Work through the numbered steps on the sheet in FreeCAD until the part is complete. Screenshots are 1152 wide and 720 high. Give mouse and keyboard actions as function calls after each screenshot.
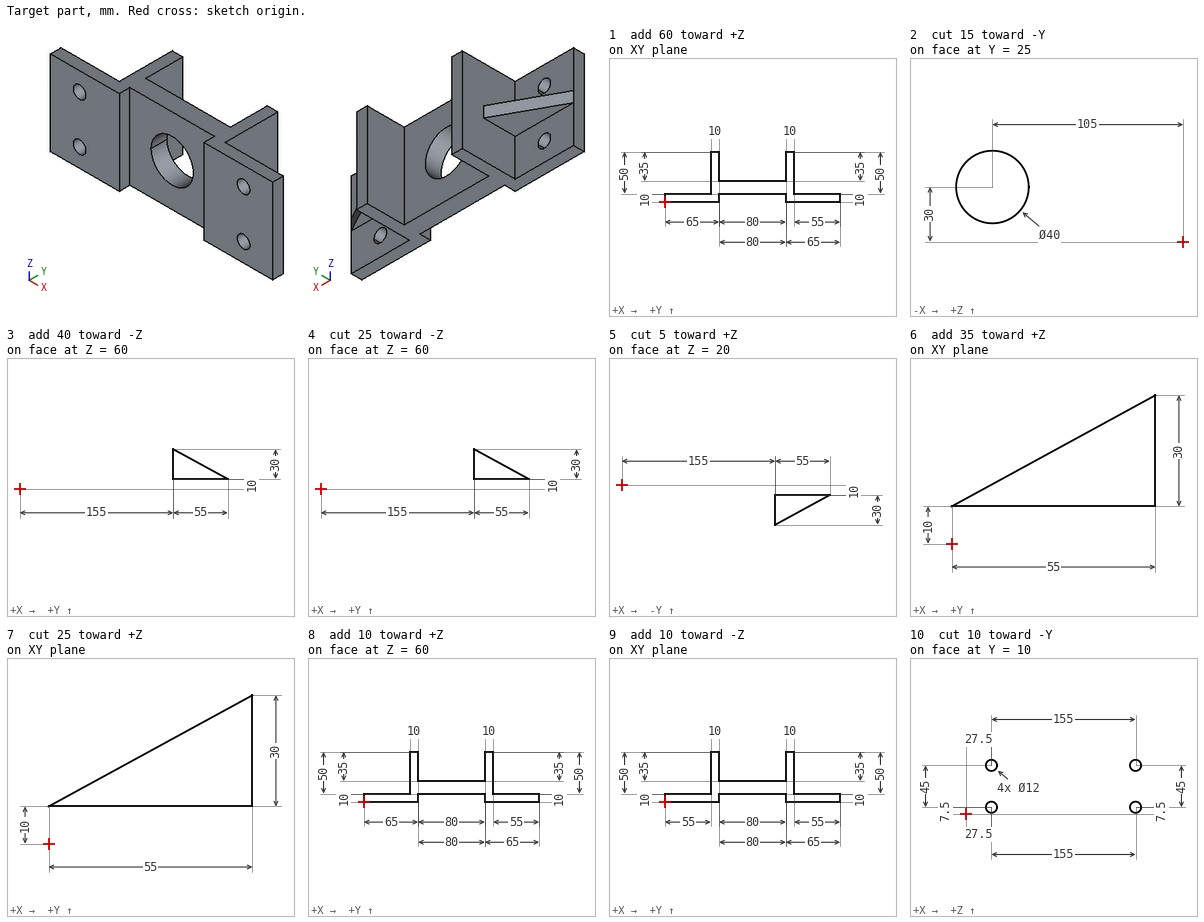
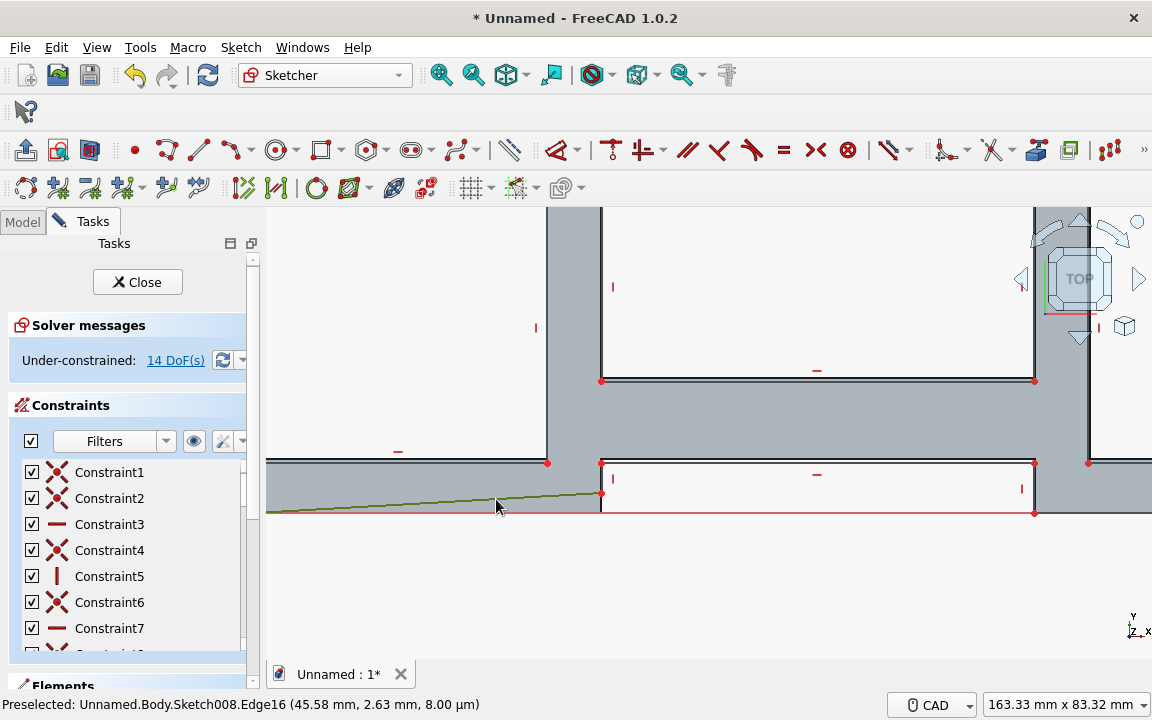
key(h)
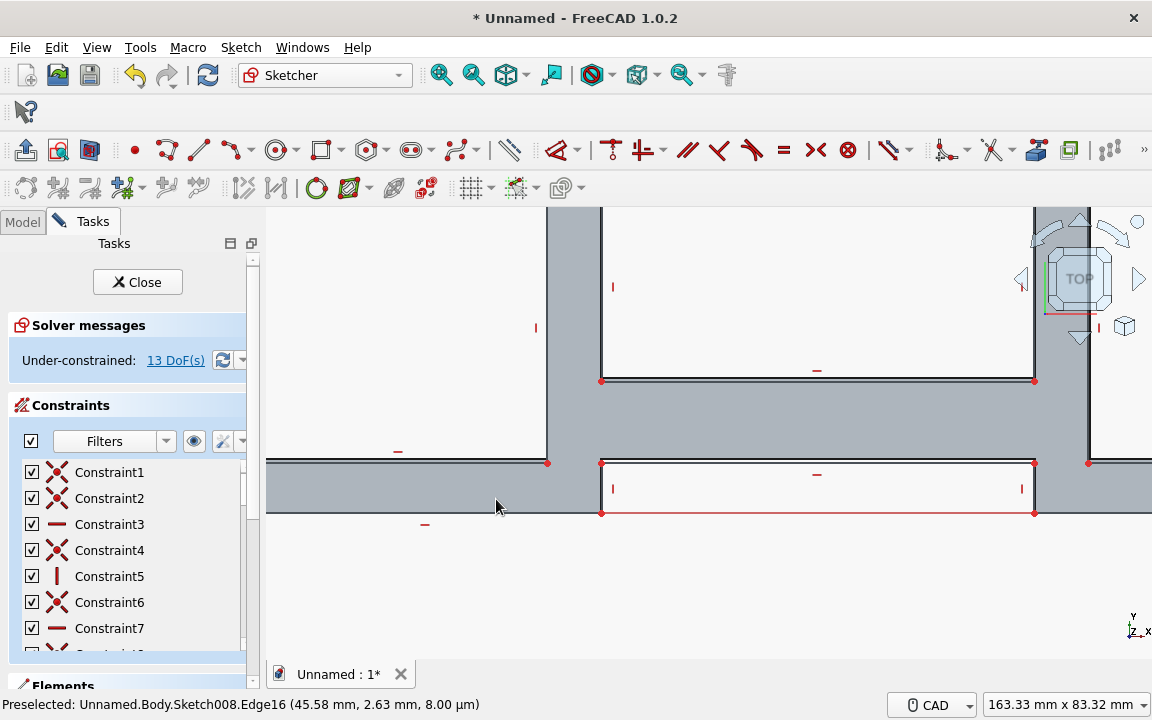
click(556, 150)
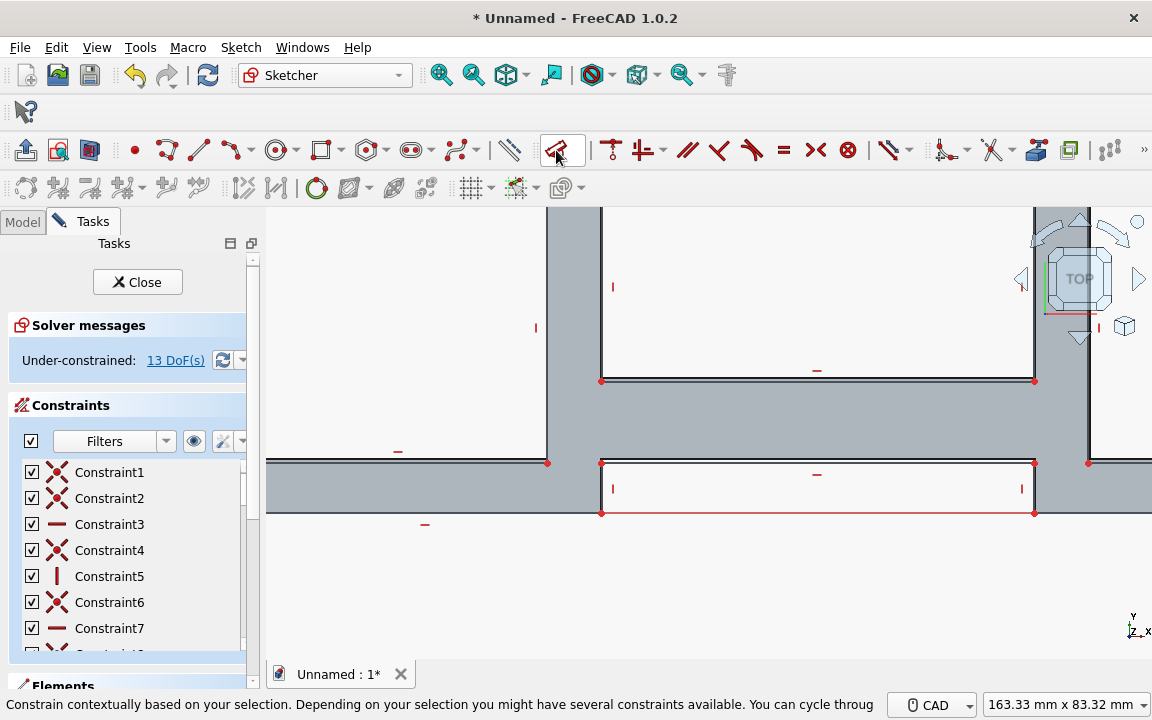
scroll(495, 500, down, 4)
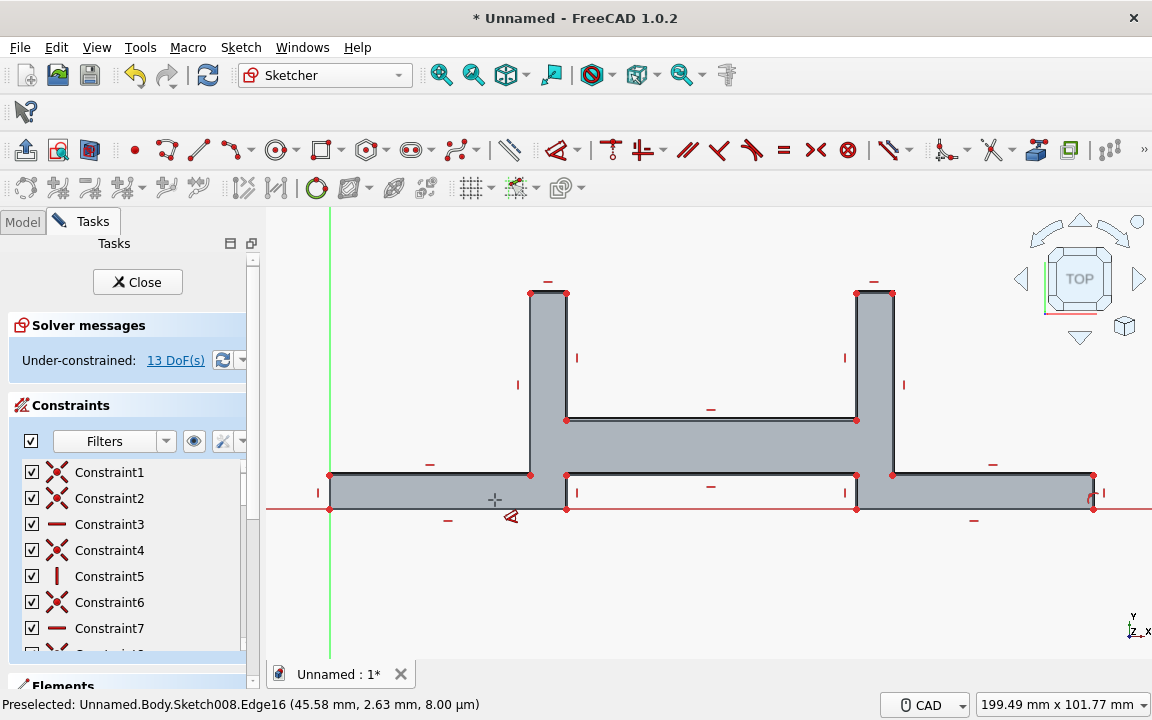
scroll(384, 500, up, 4)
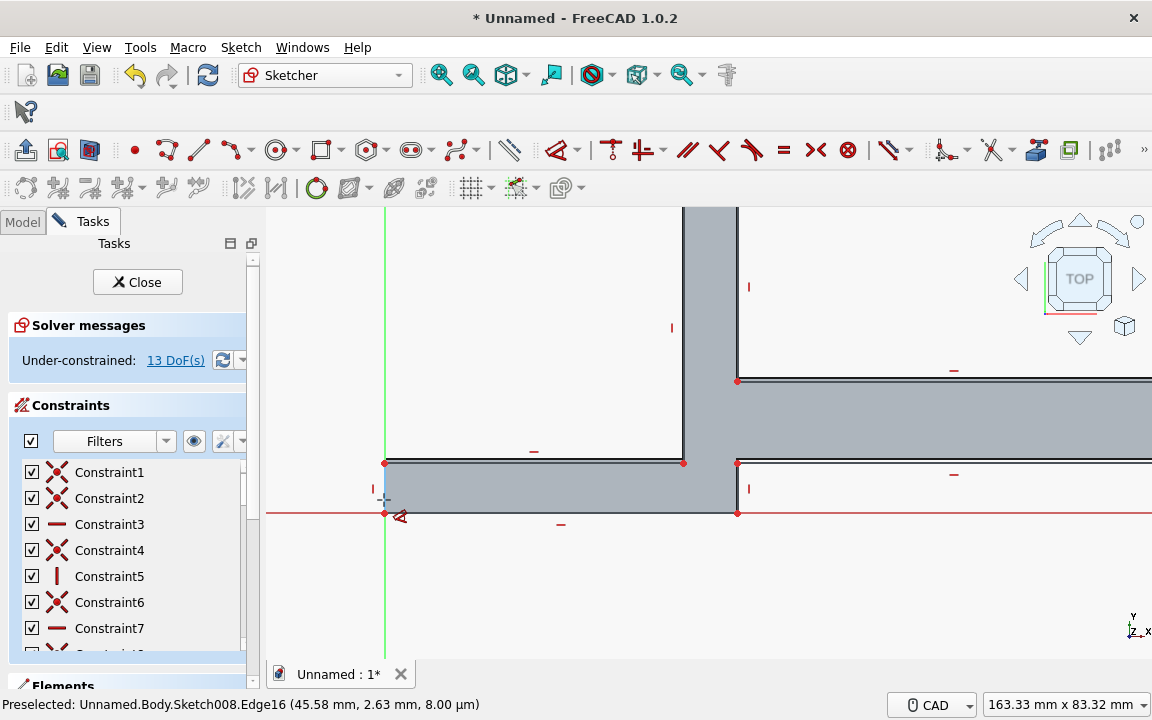
click(385, 498)
click(351, 488)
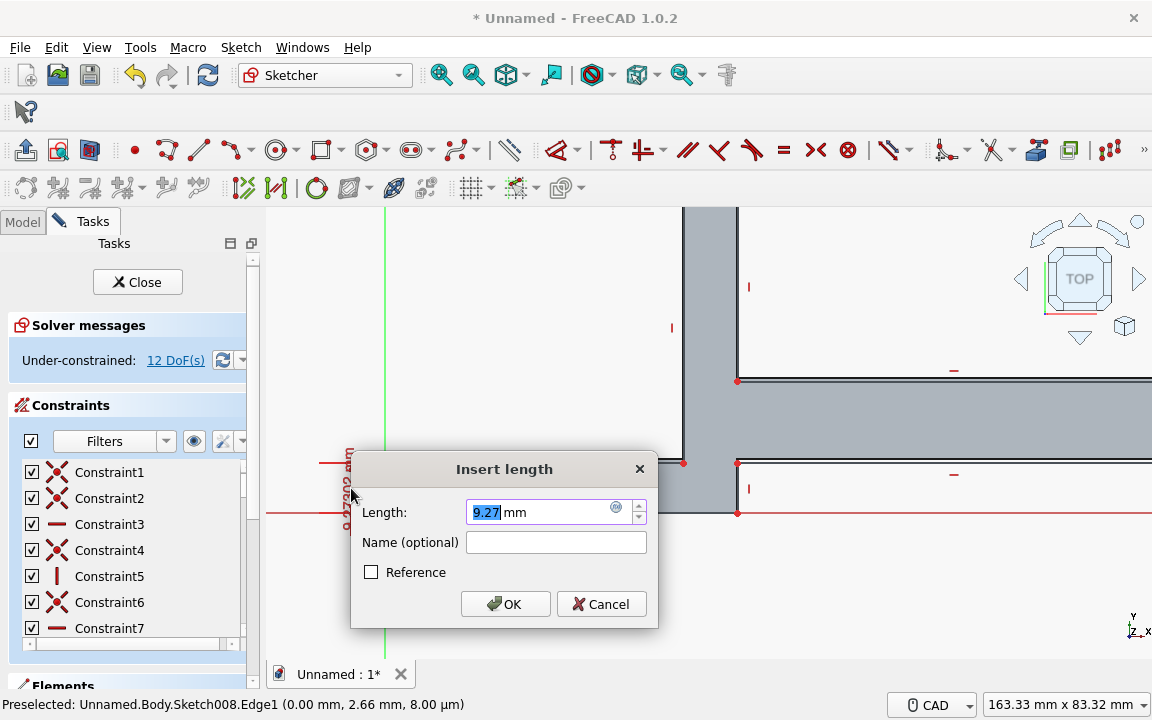
text(10)
key(Return)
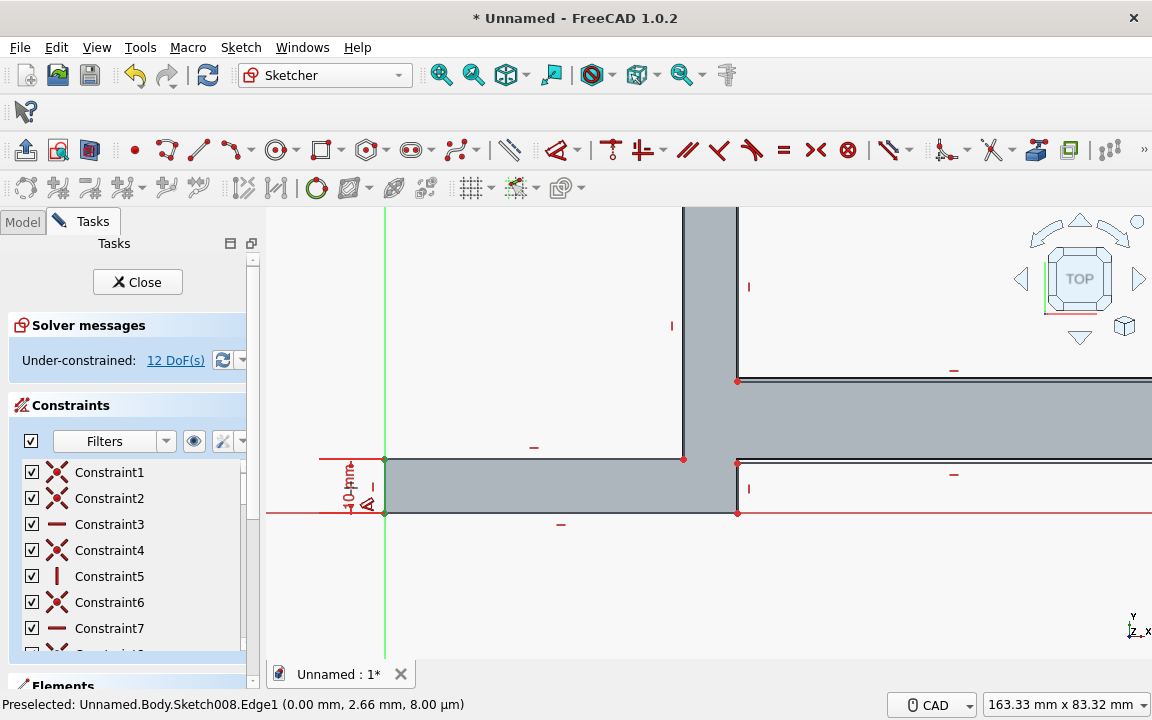
click(475, 459)
click(534, 493)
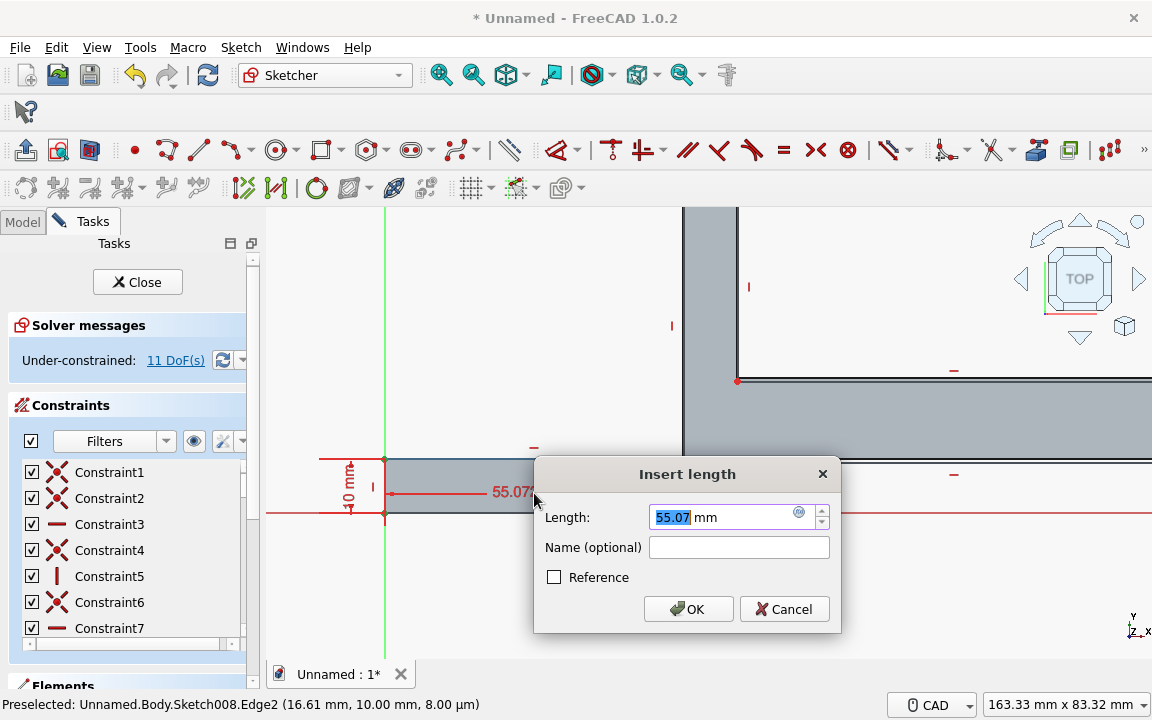
text(55)
key(Return)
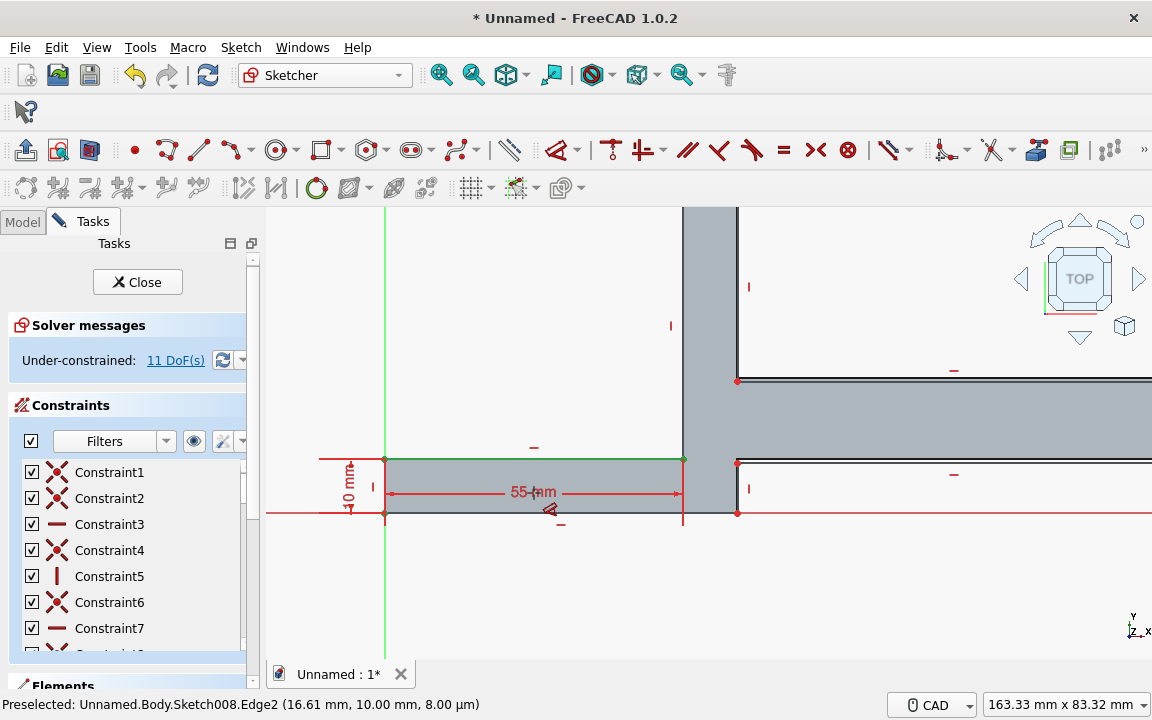
click(683, 379)
click(649, 347)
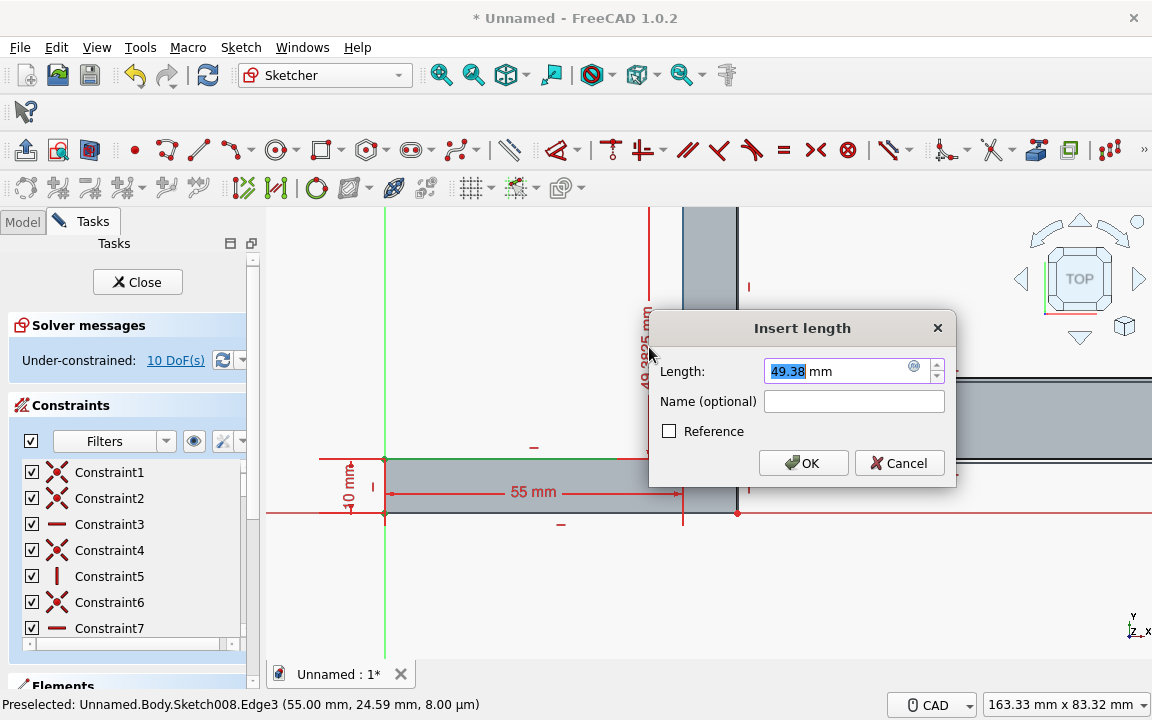
text(50)
key(Return)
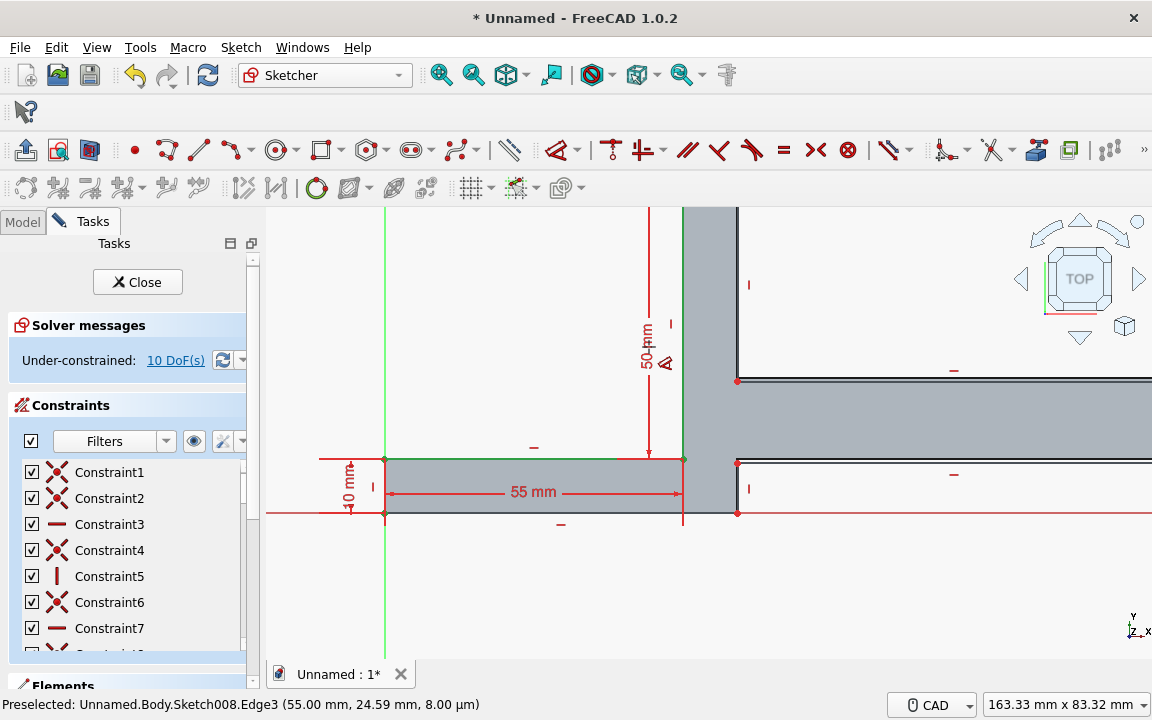
scroll(384, 500, down, 4)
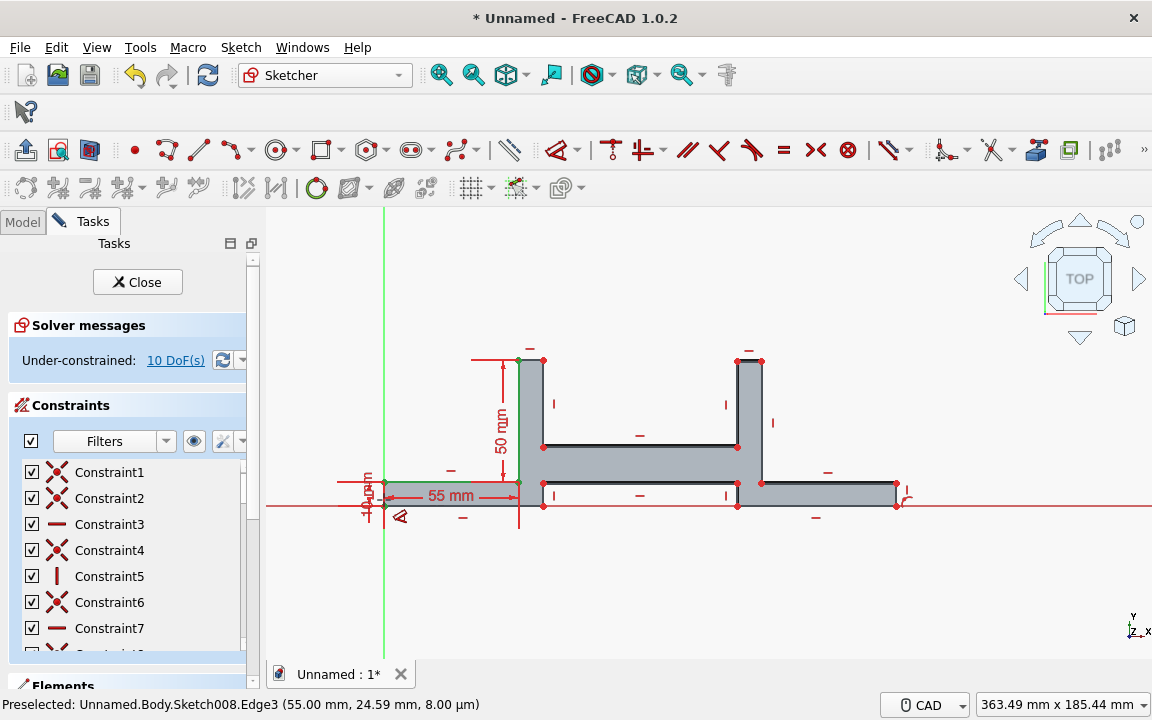
scroll(526, 360, up, 4)